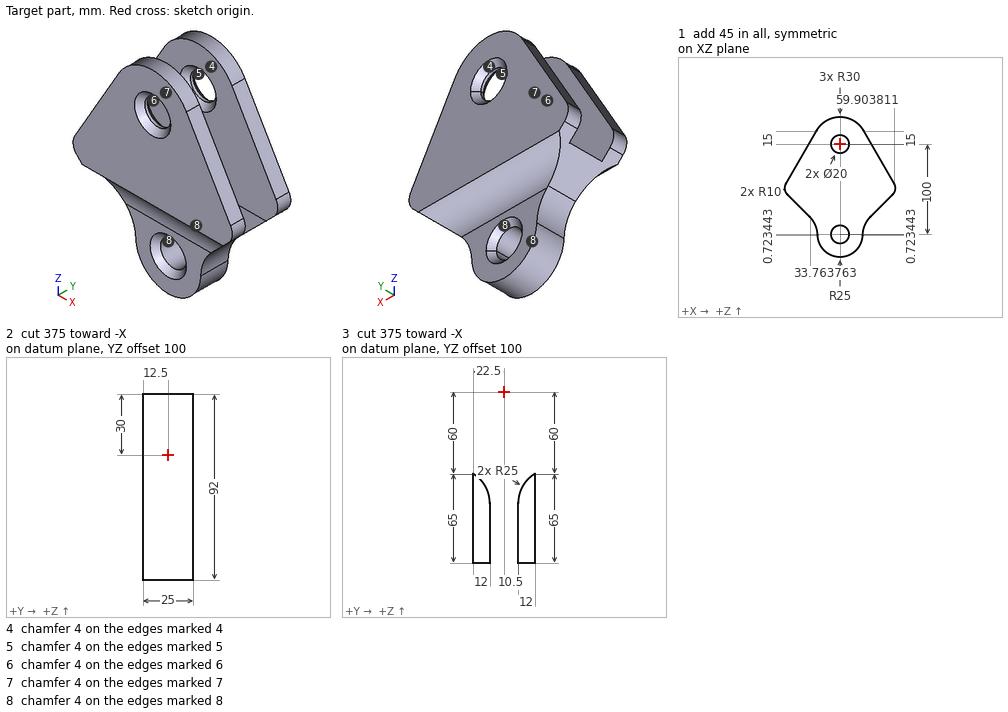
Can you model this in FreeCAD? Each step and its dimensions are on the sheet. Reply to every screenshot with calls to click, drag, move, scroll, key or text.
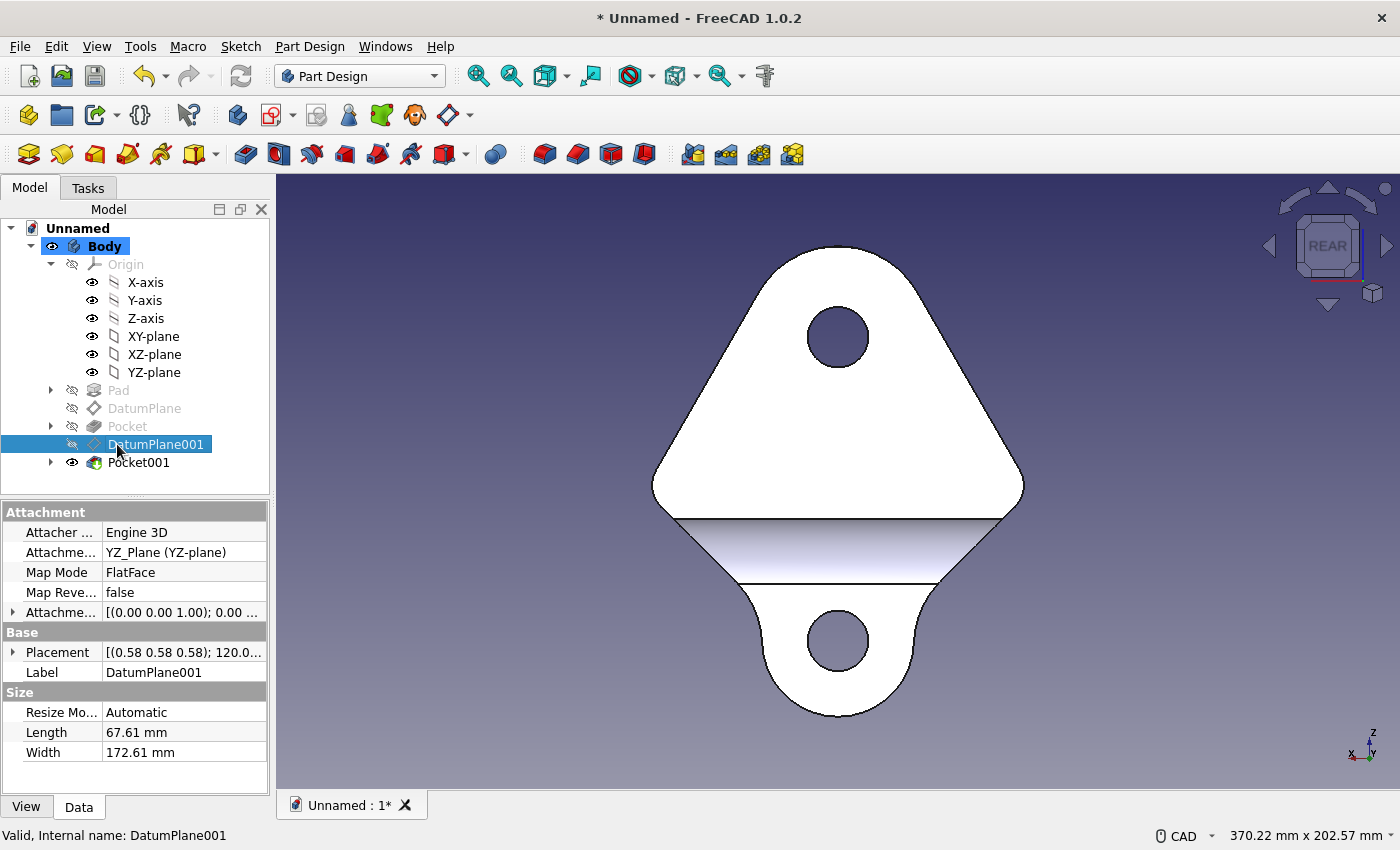
click(863, 318)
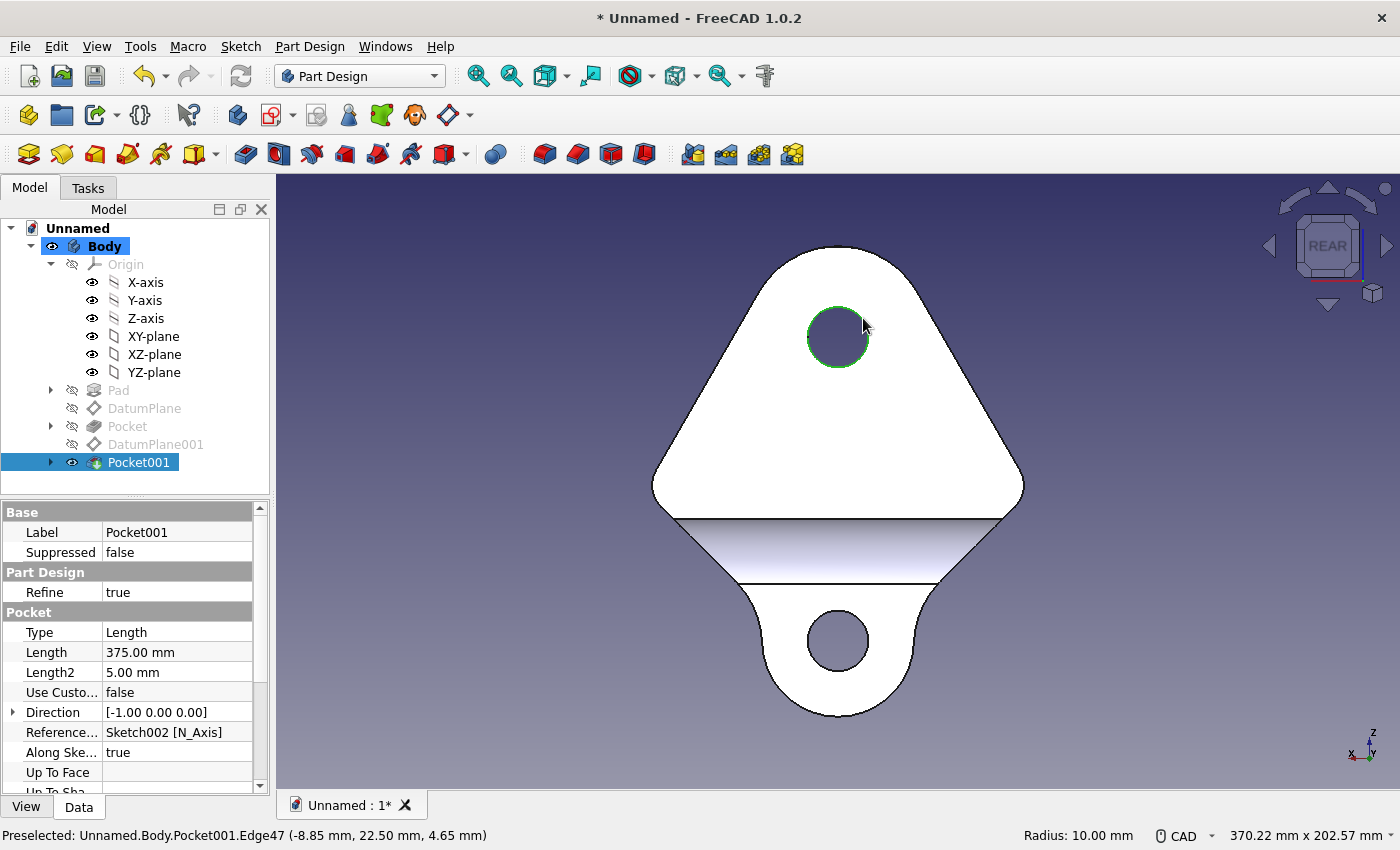
click(578, 154)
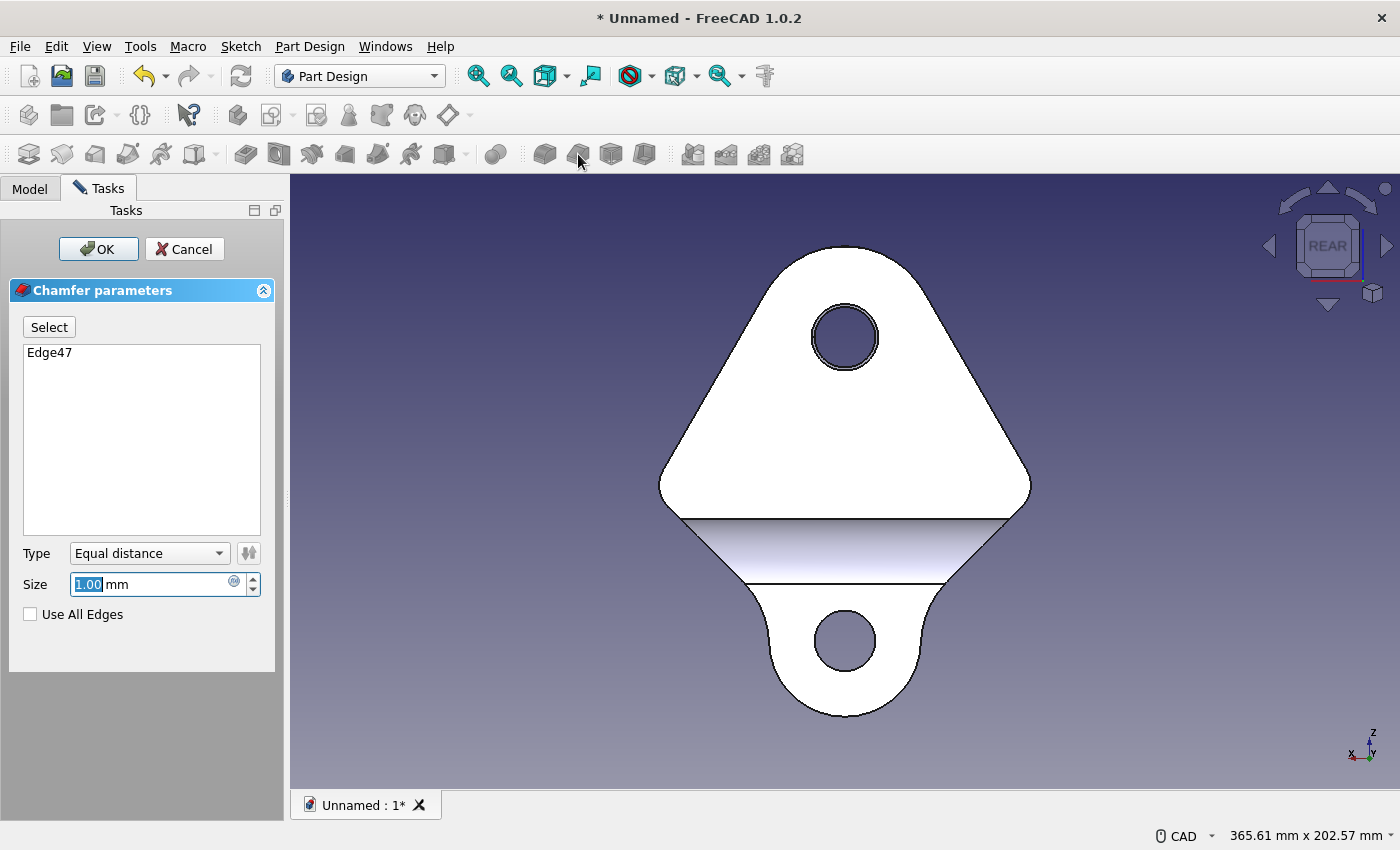
text(4)
key(Tab)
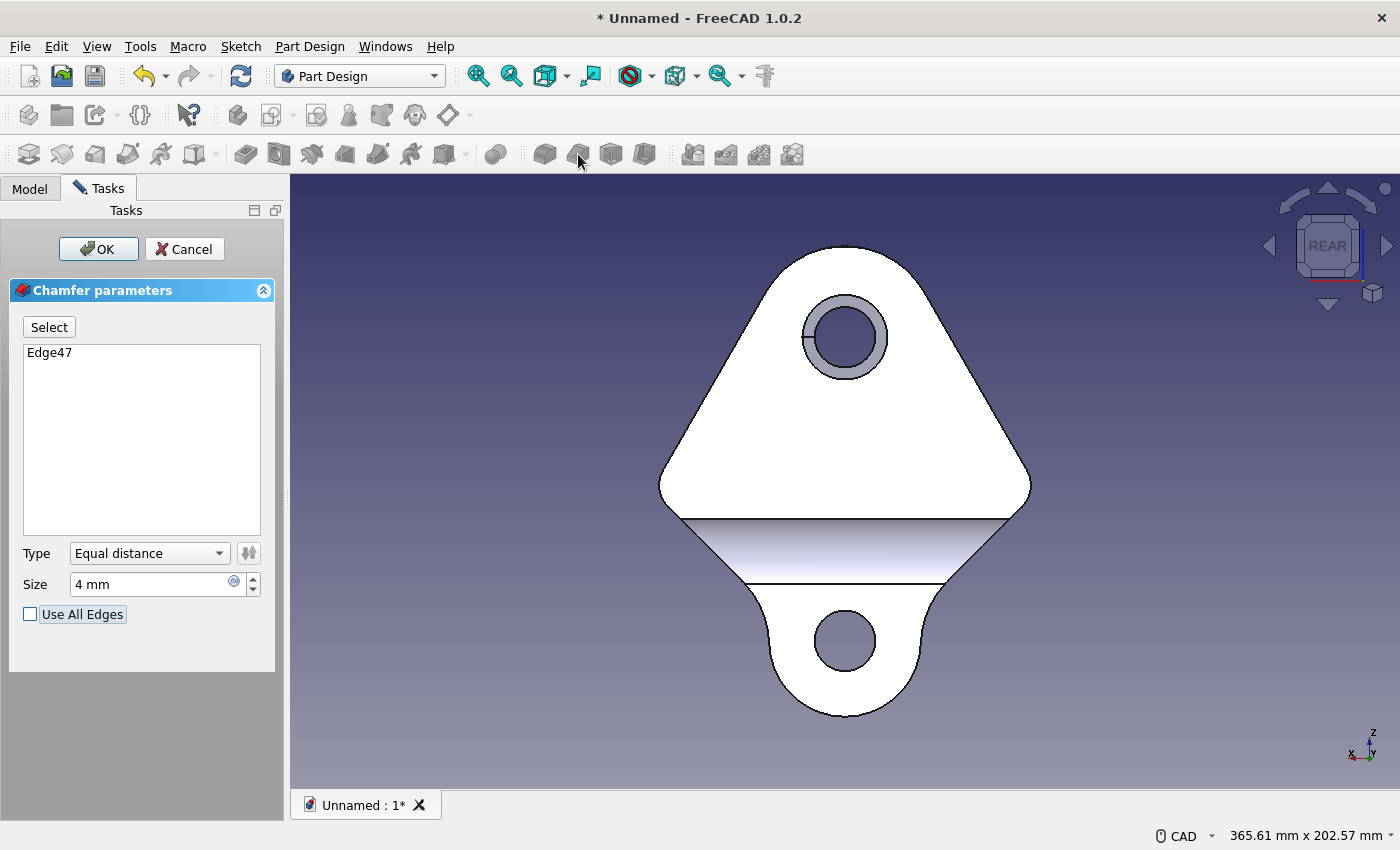
click(99, 249)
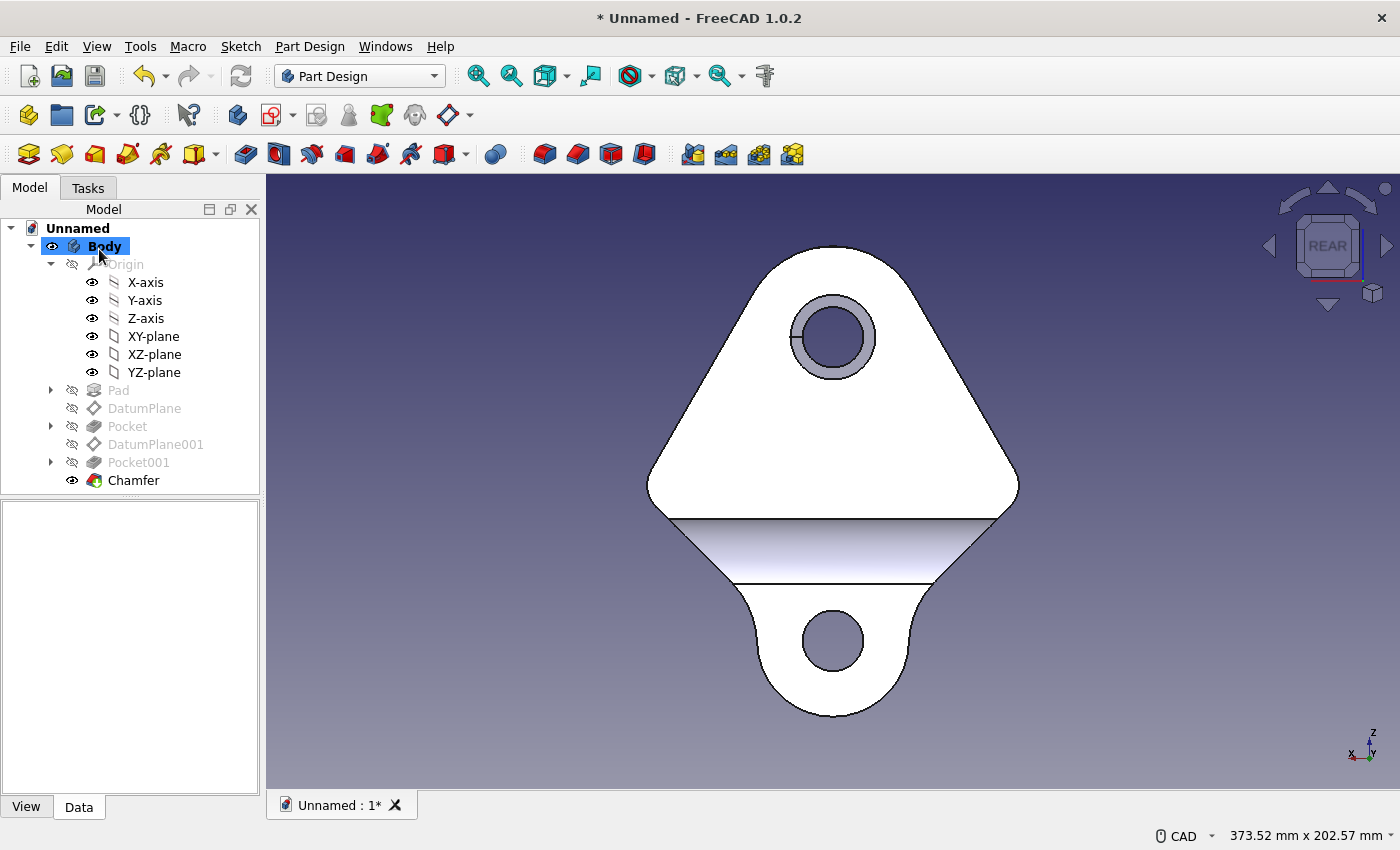
key(0)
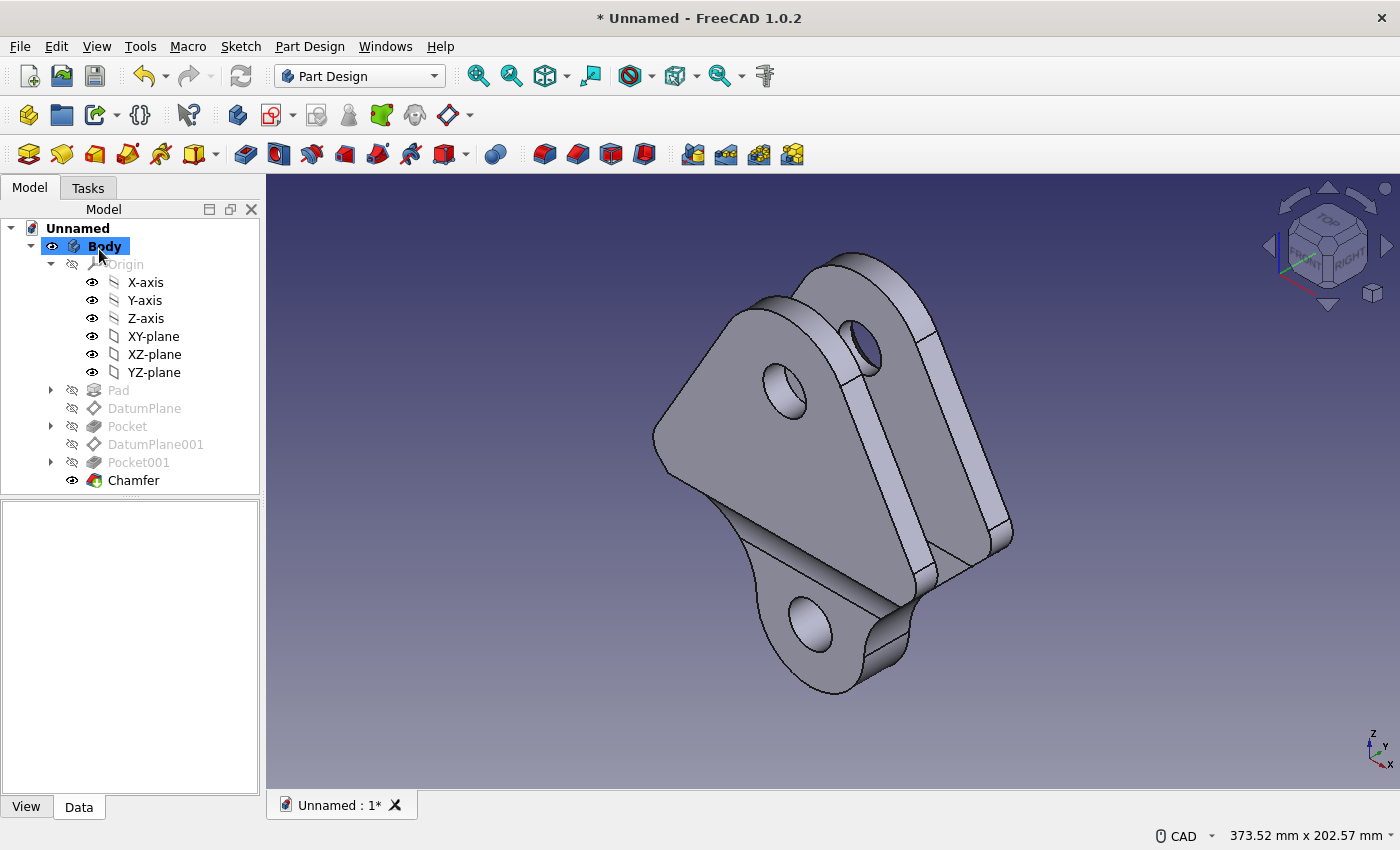
click(842, 323)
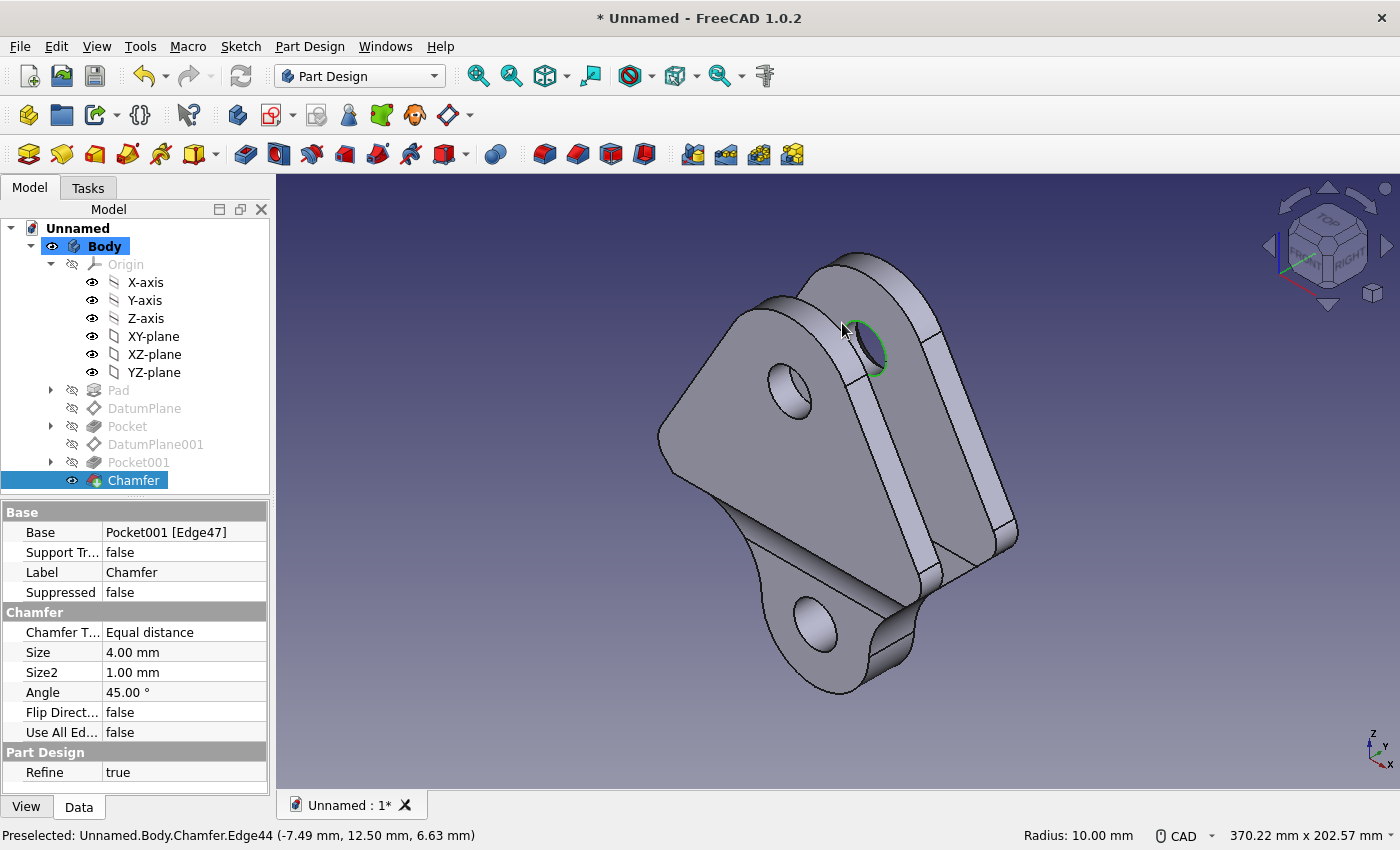
click(578, 154)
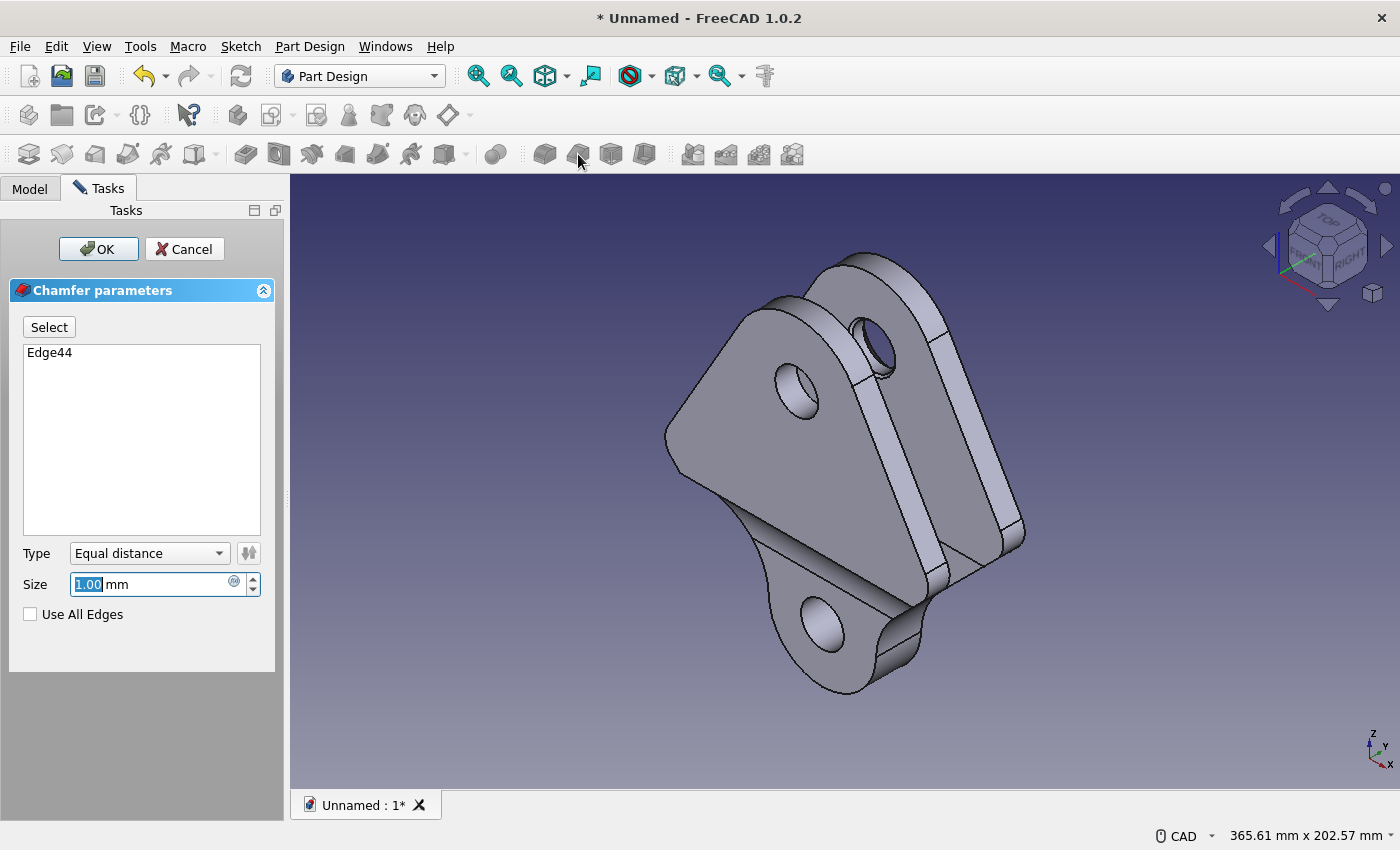
text(4)
key(Tab)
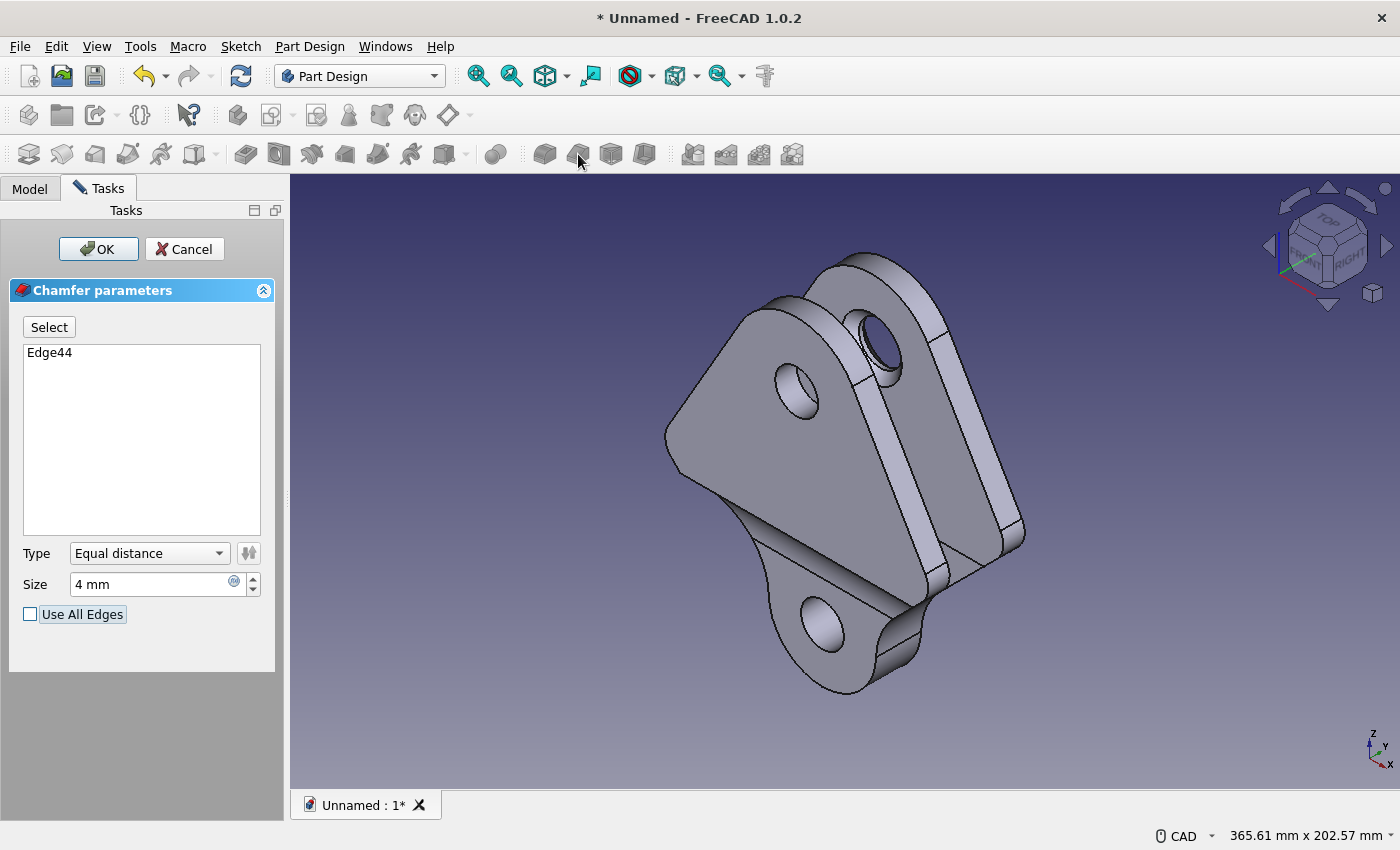
click(99, 249)